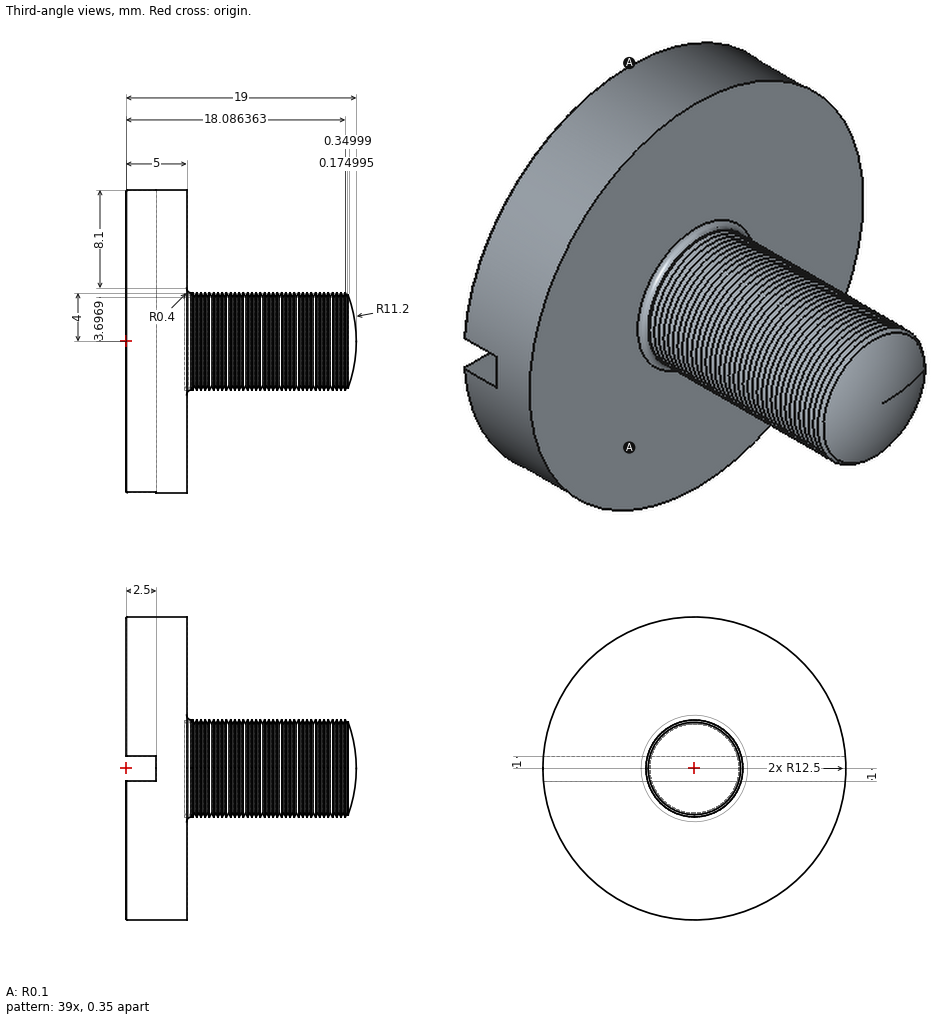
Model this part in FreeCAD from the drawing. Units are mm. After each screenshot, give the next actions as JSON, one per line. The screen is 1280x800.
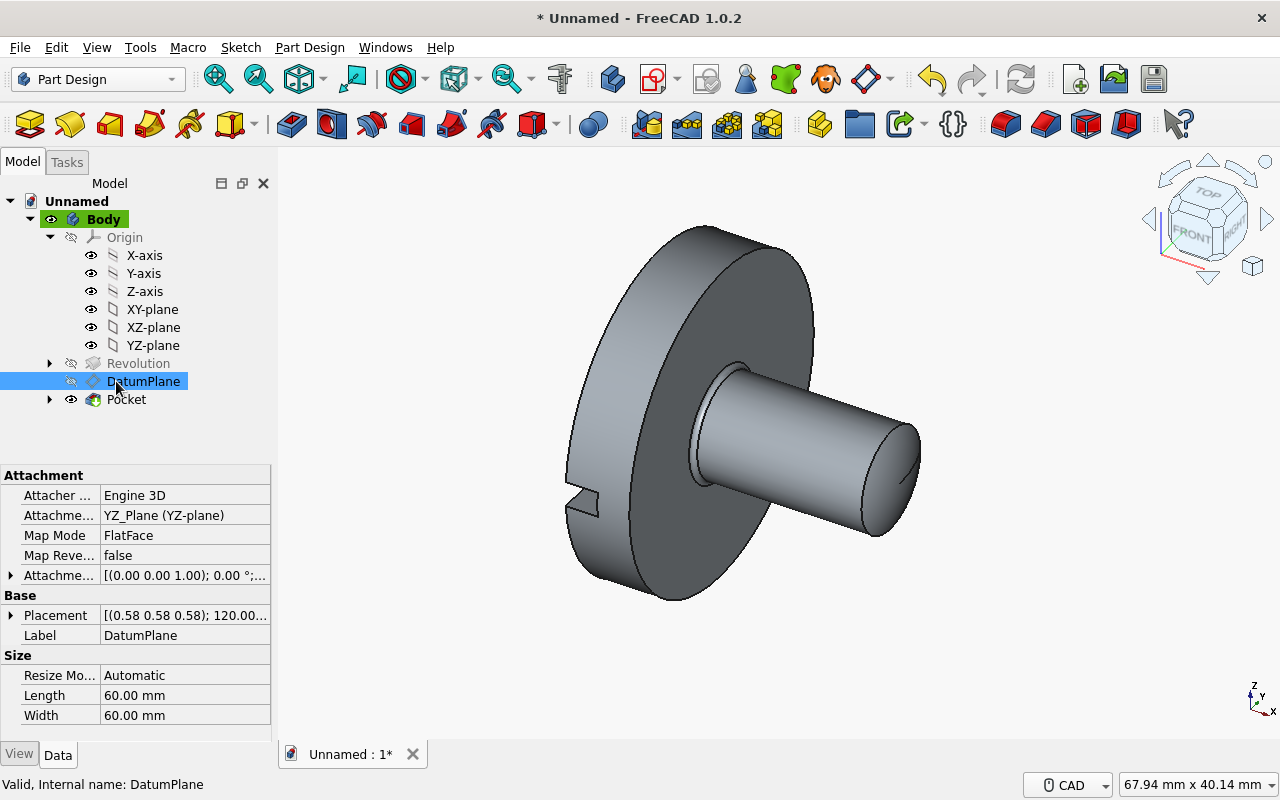
{"action": "key", "text": "0"}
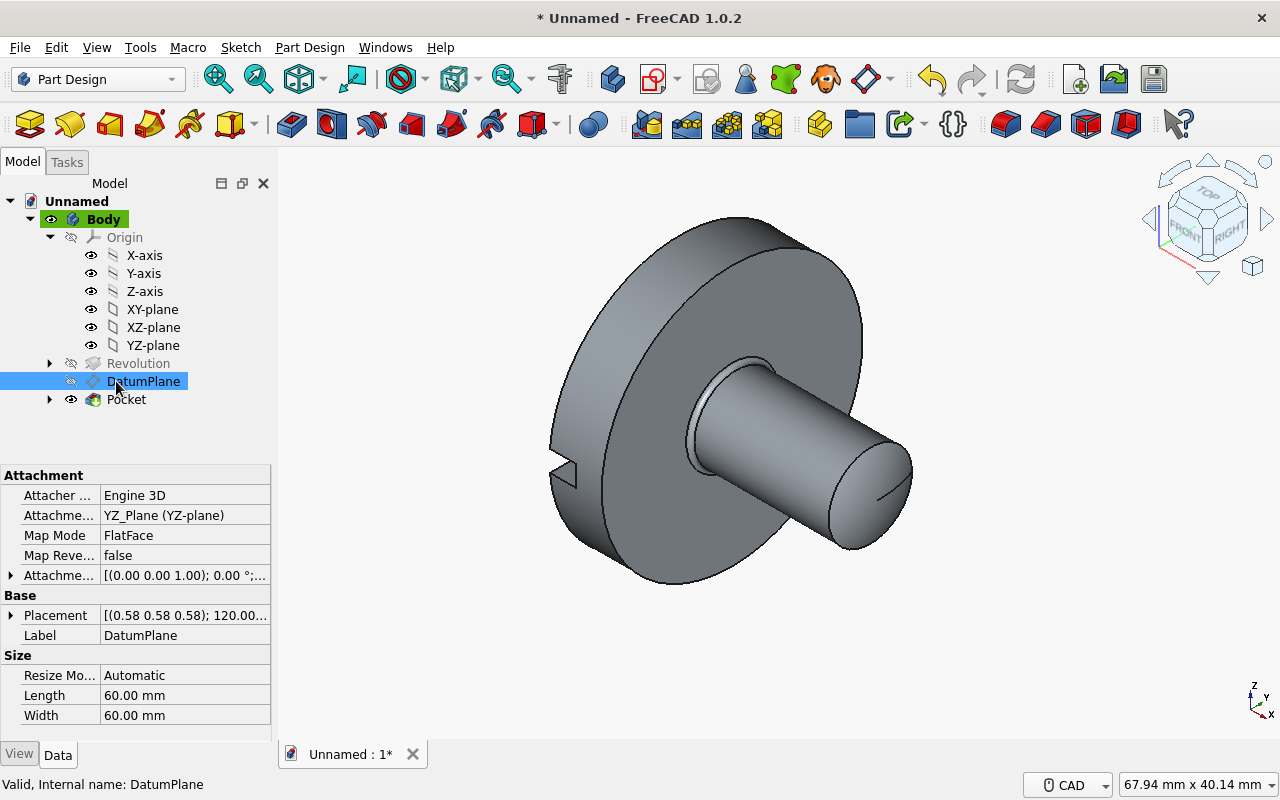
{"action": "key", "text": "2"}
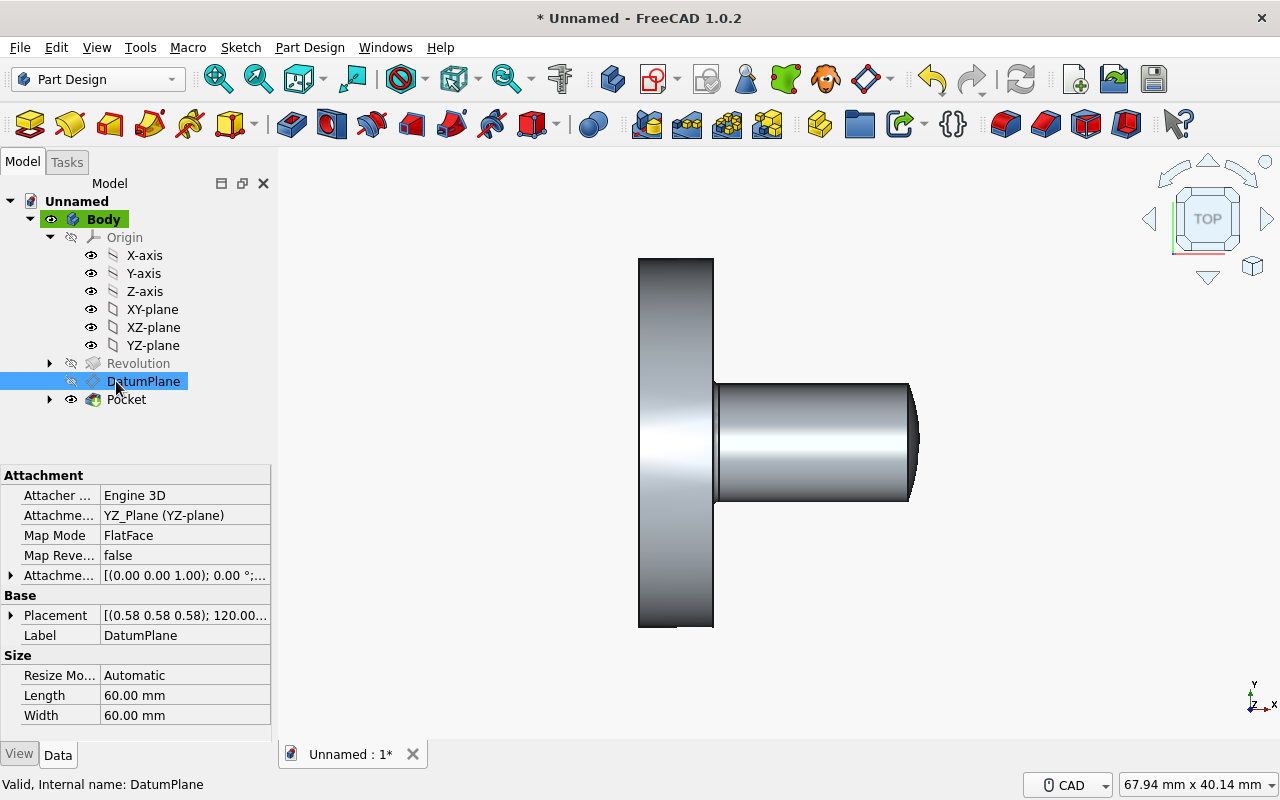
{"action": "left_click", "coordinate": [639, 260]}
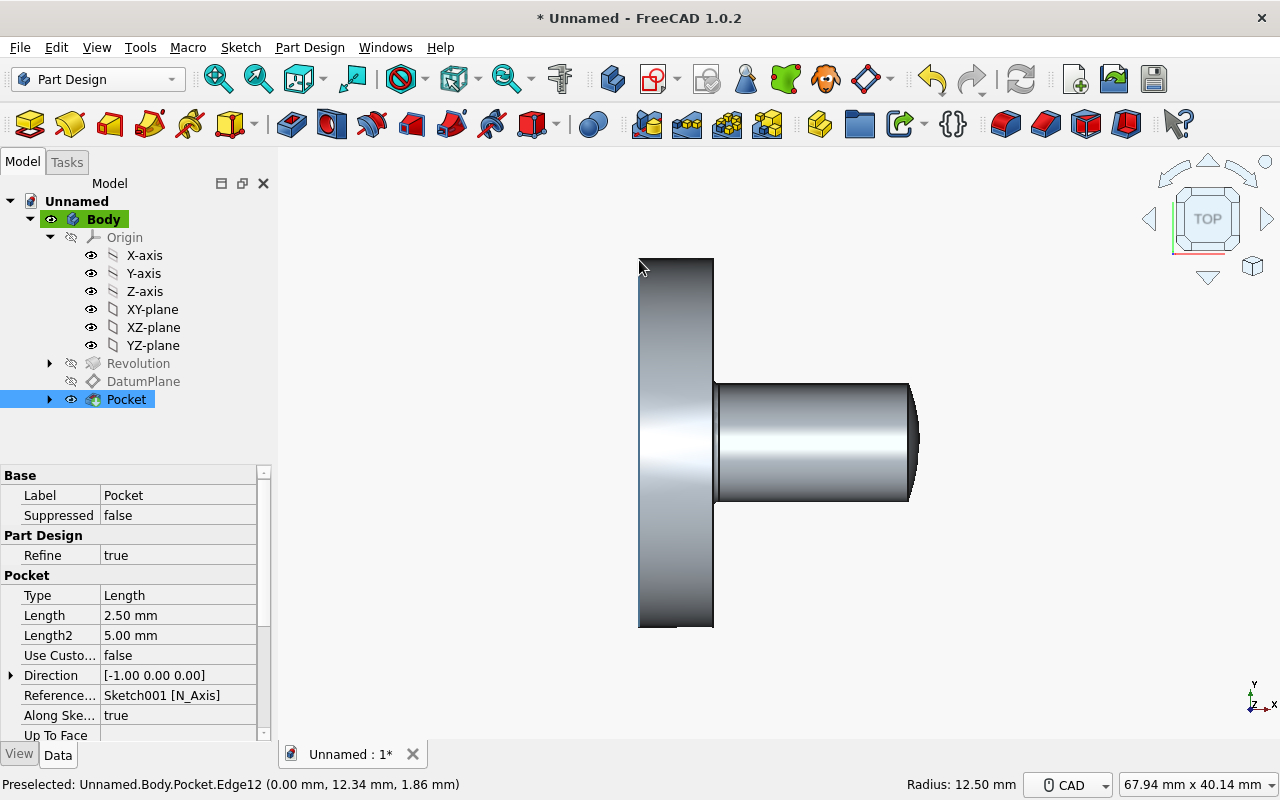
{"action": "key", "text": "1"}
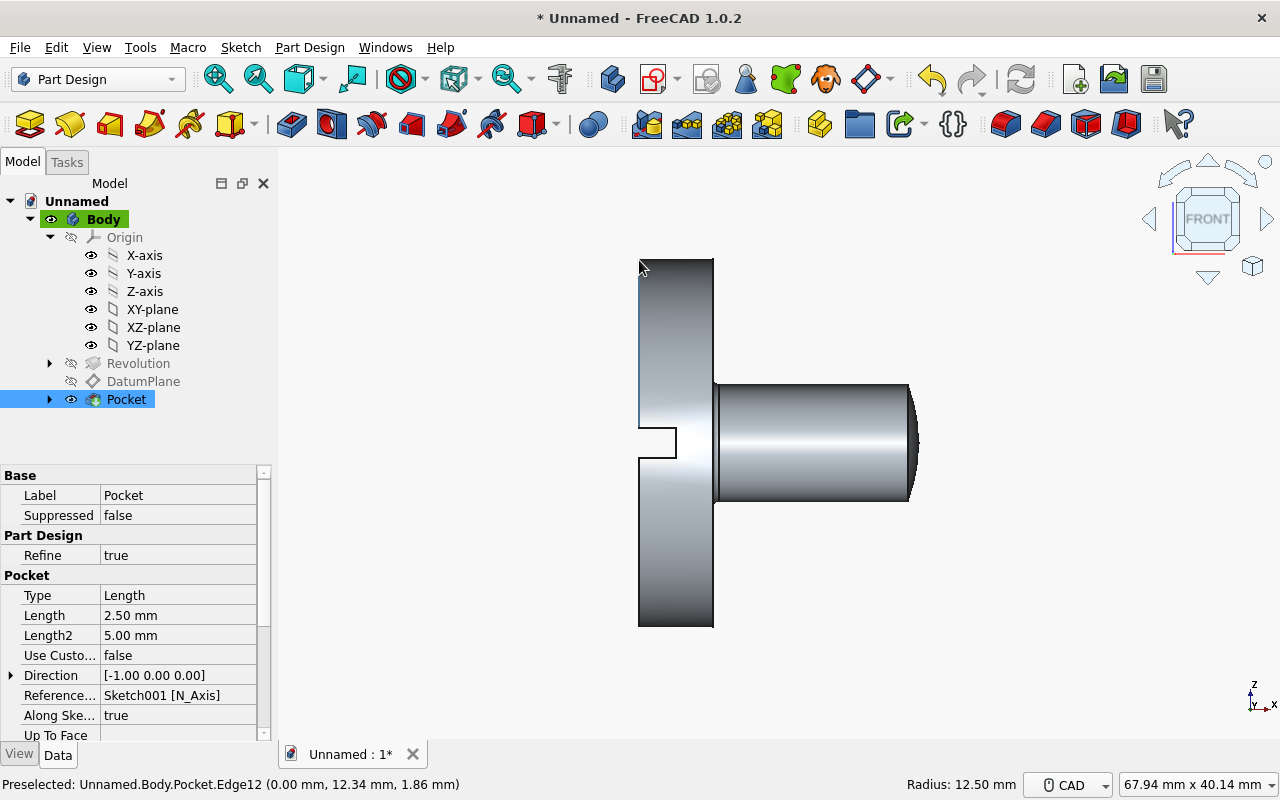
{"action": "left_click", "coordinate": [639, 473], "text": "ctrl"}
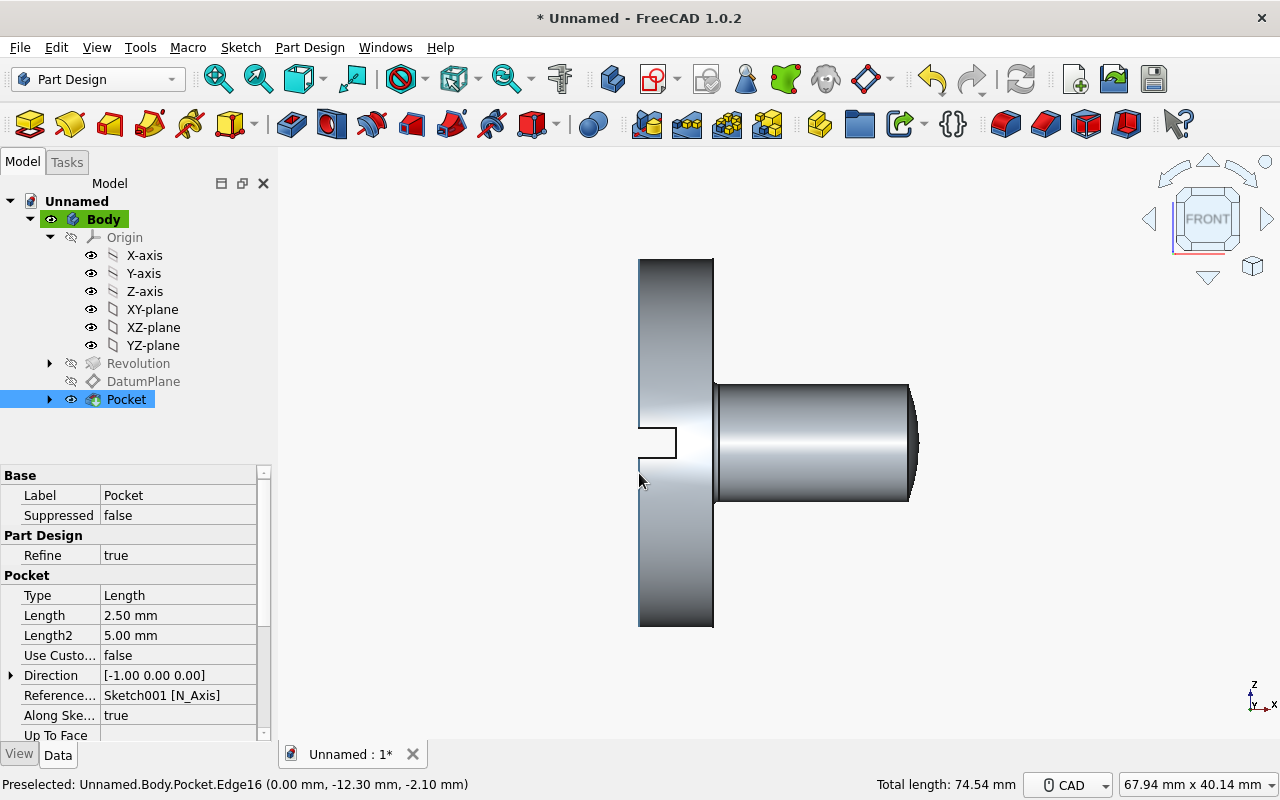
{"action": "left_click", "coordinate": [1006, 124]}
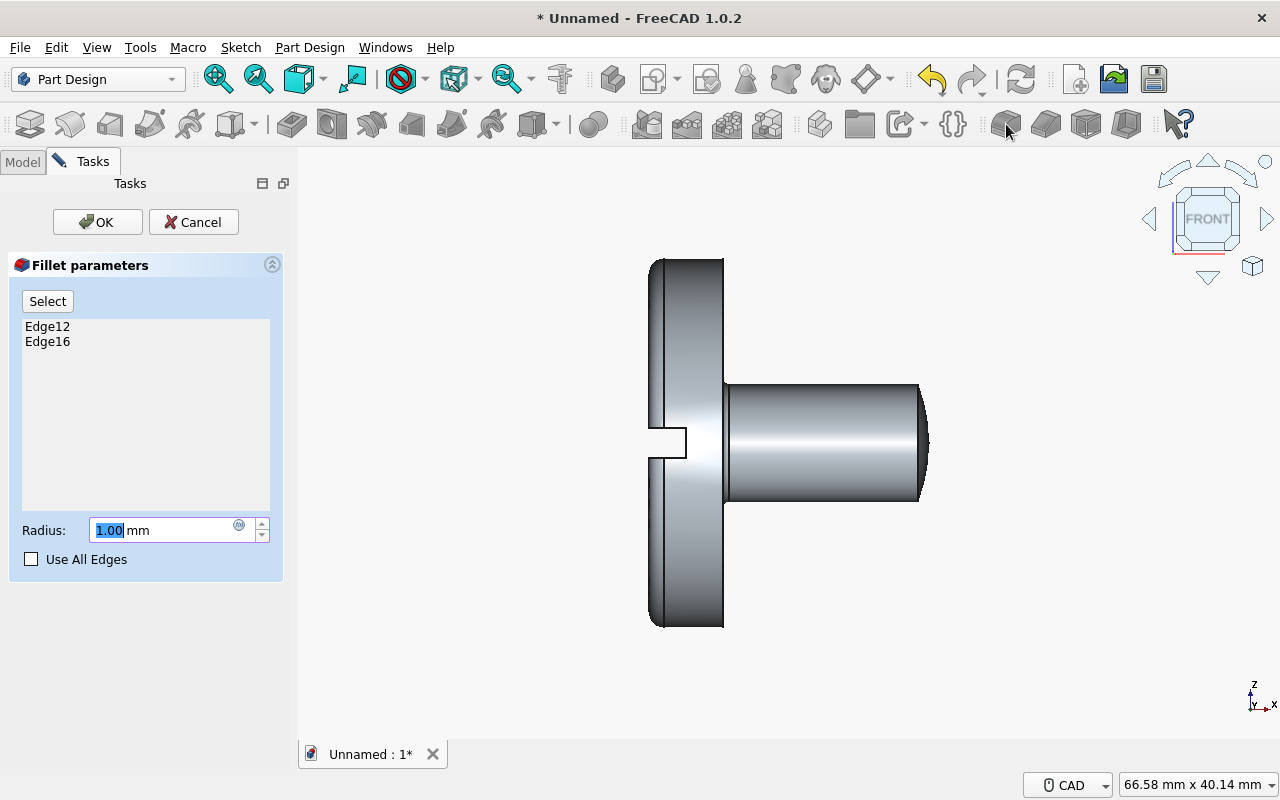
{"action": "type", "text": "0.1"}
{"action": "key", "text": "Tab"}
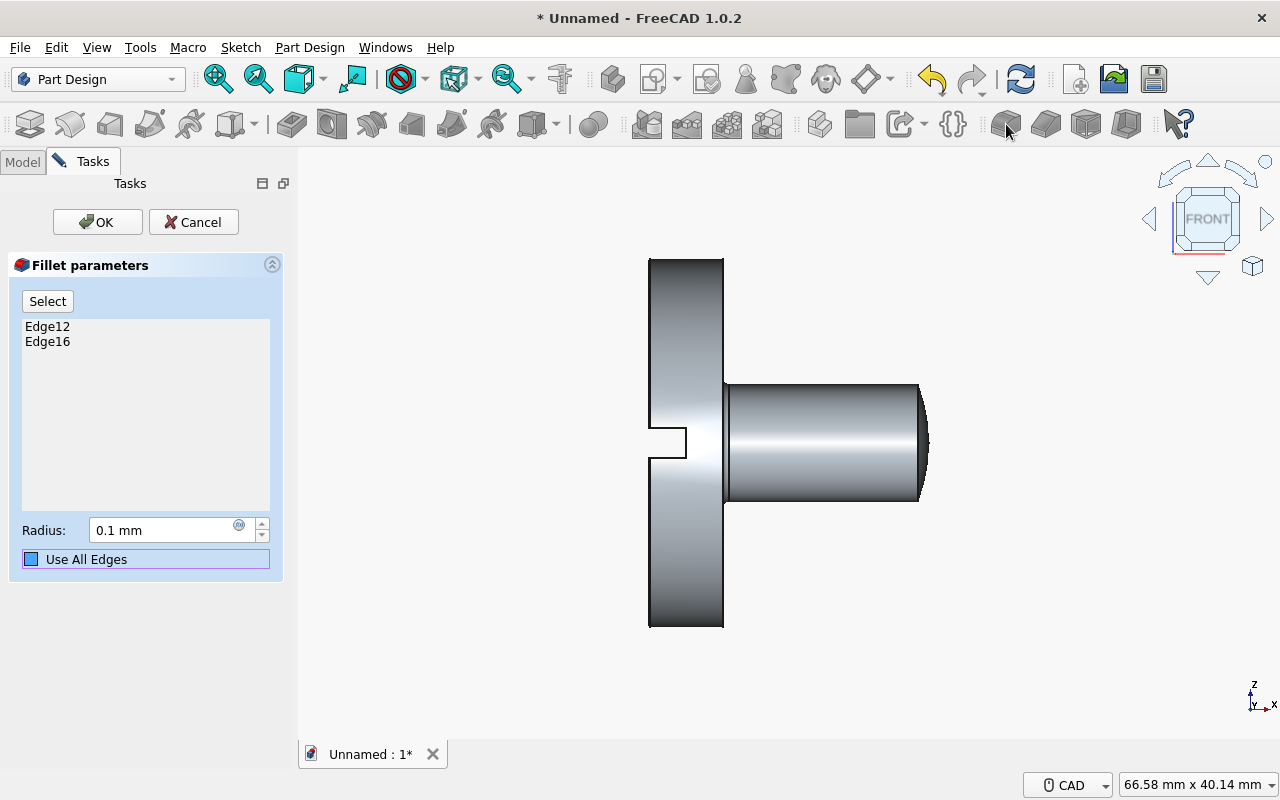
{"action": "left_click", "coordinate": [98, 222]}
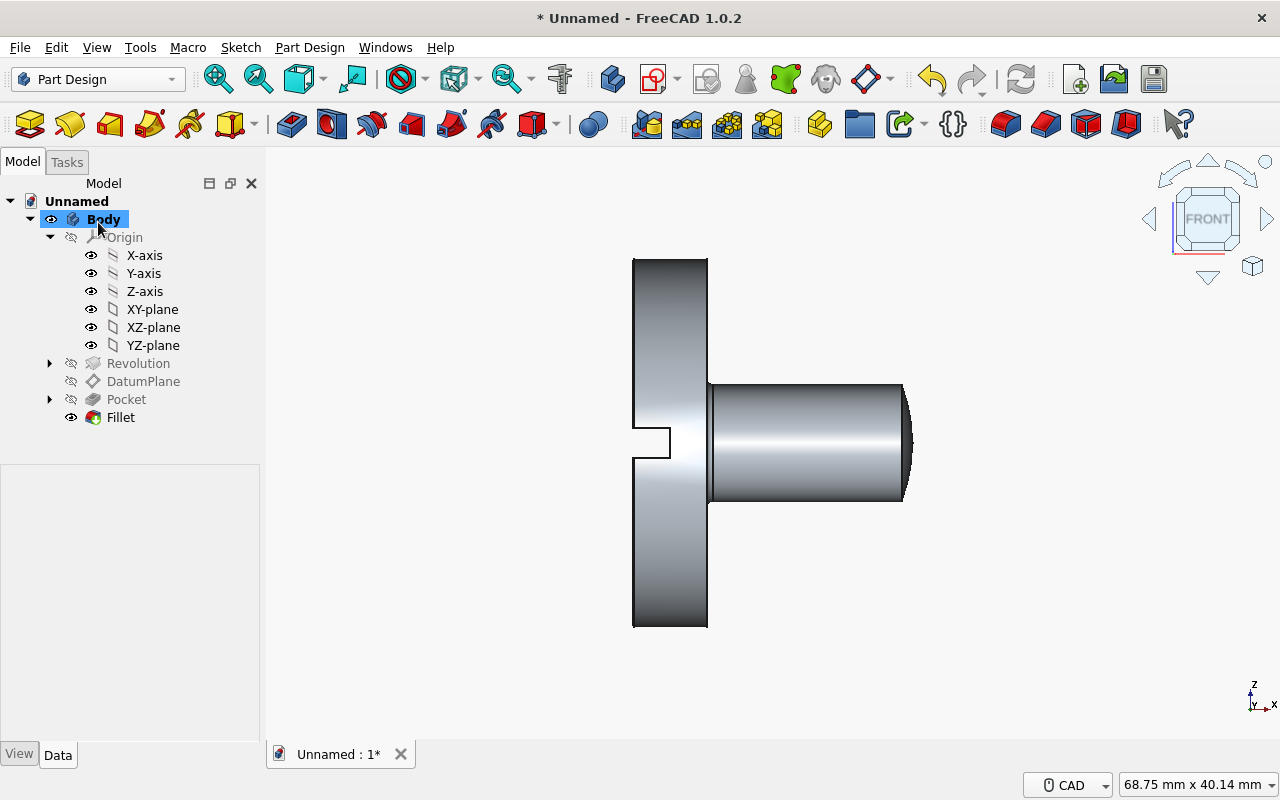
{"action": "left_click", "coordinate": [654, 80]}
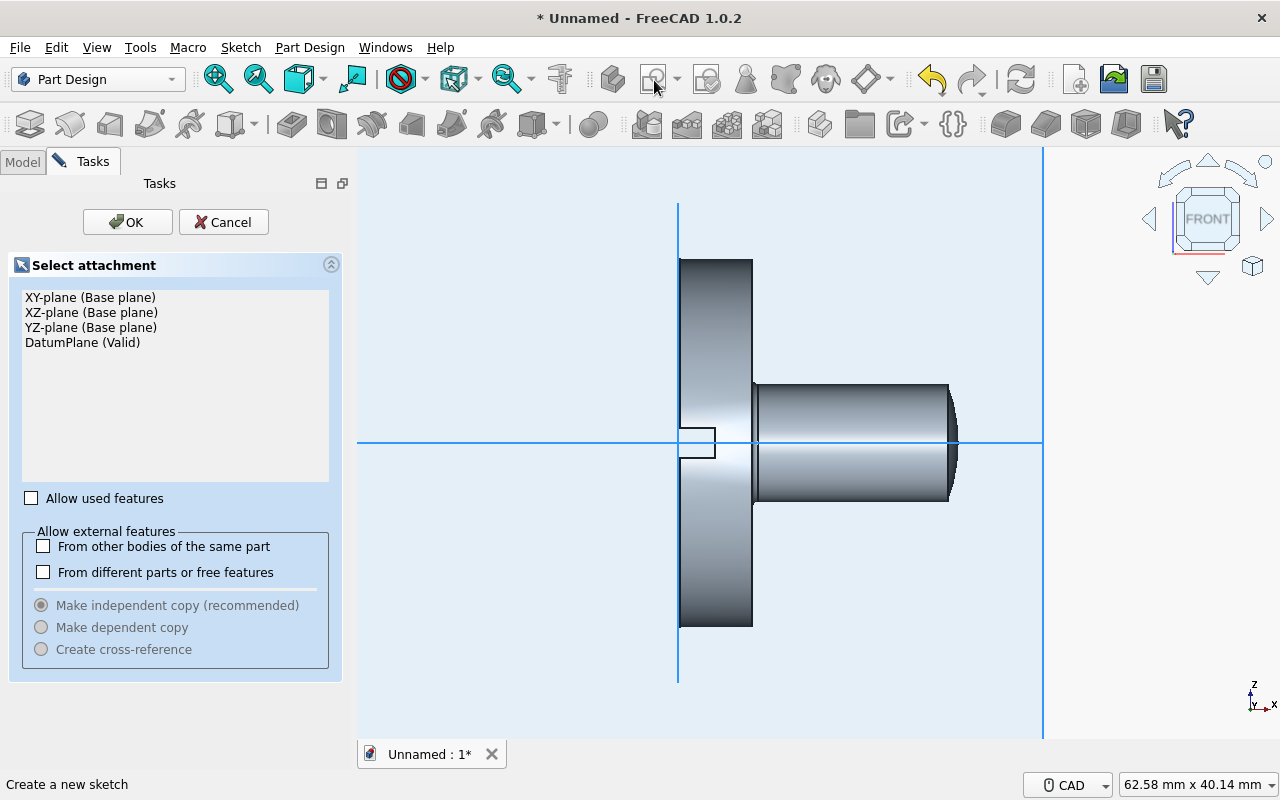
{"action": "left_click", "coordinate": [82, 298]}